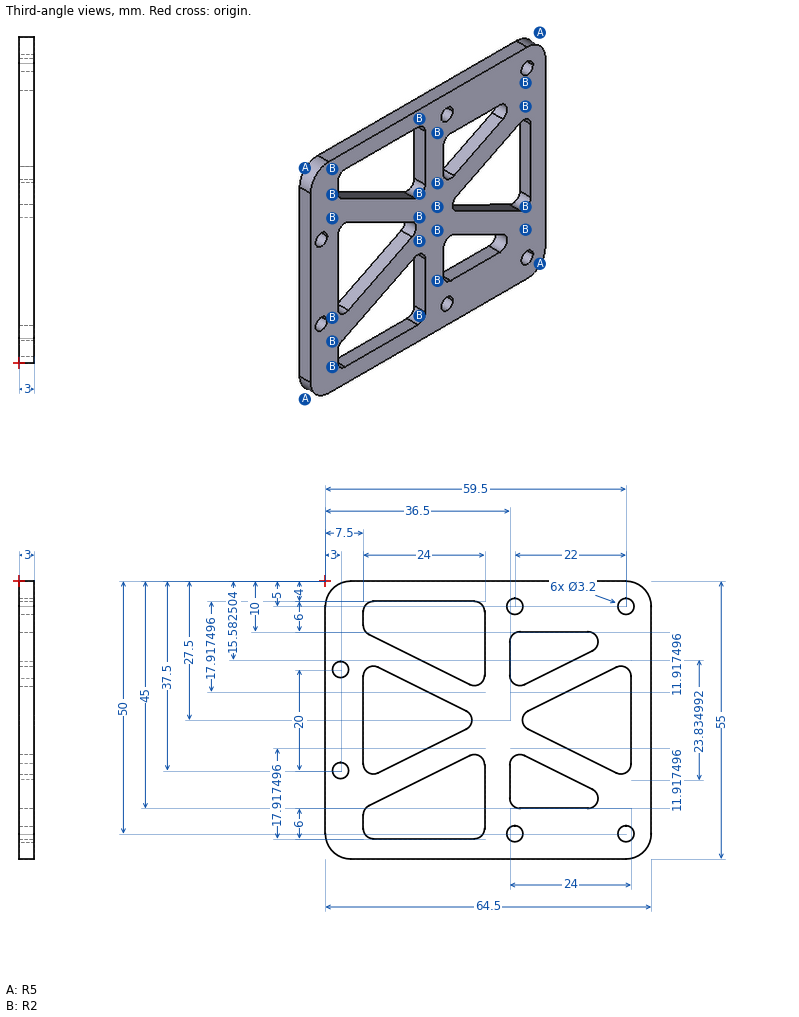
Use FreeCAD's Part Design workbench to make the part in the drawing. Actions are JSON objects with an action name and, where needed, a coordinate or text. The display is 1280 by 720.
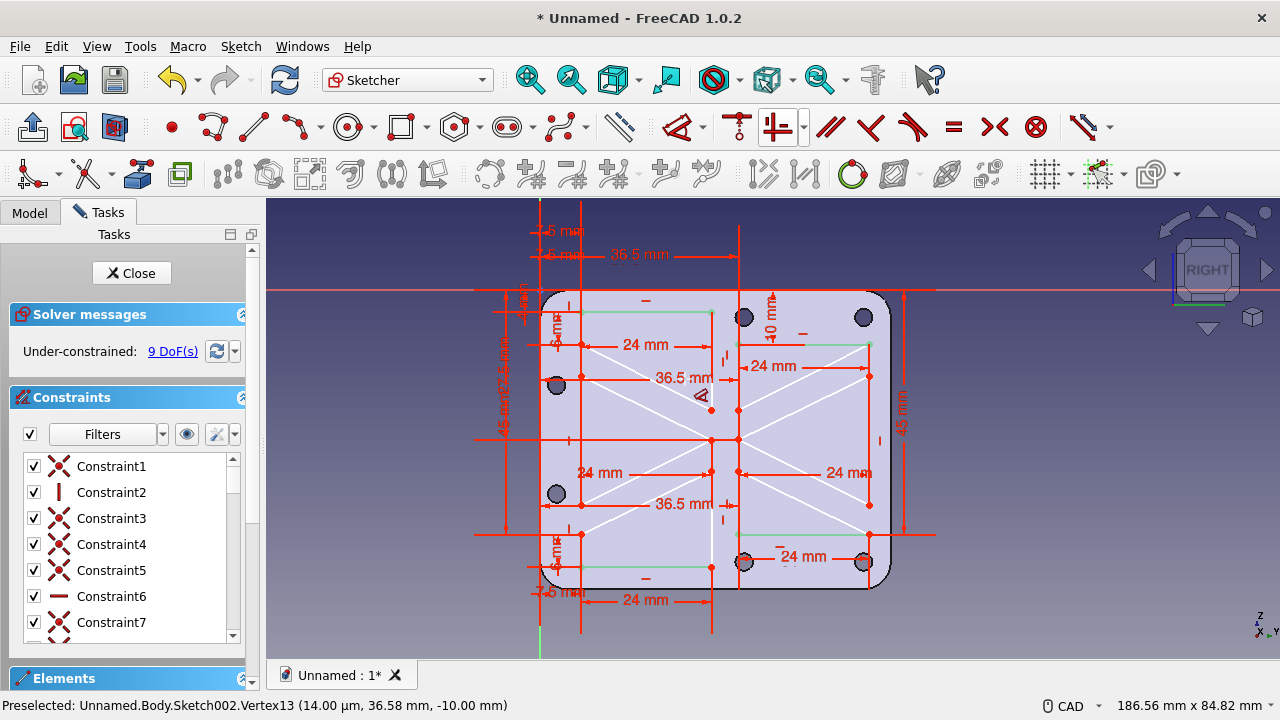
{"action": "left_click", "coordinate": [712, 440]}
{"action": "left_click", "coordinate": [482, 331]}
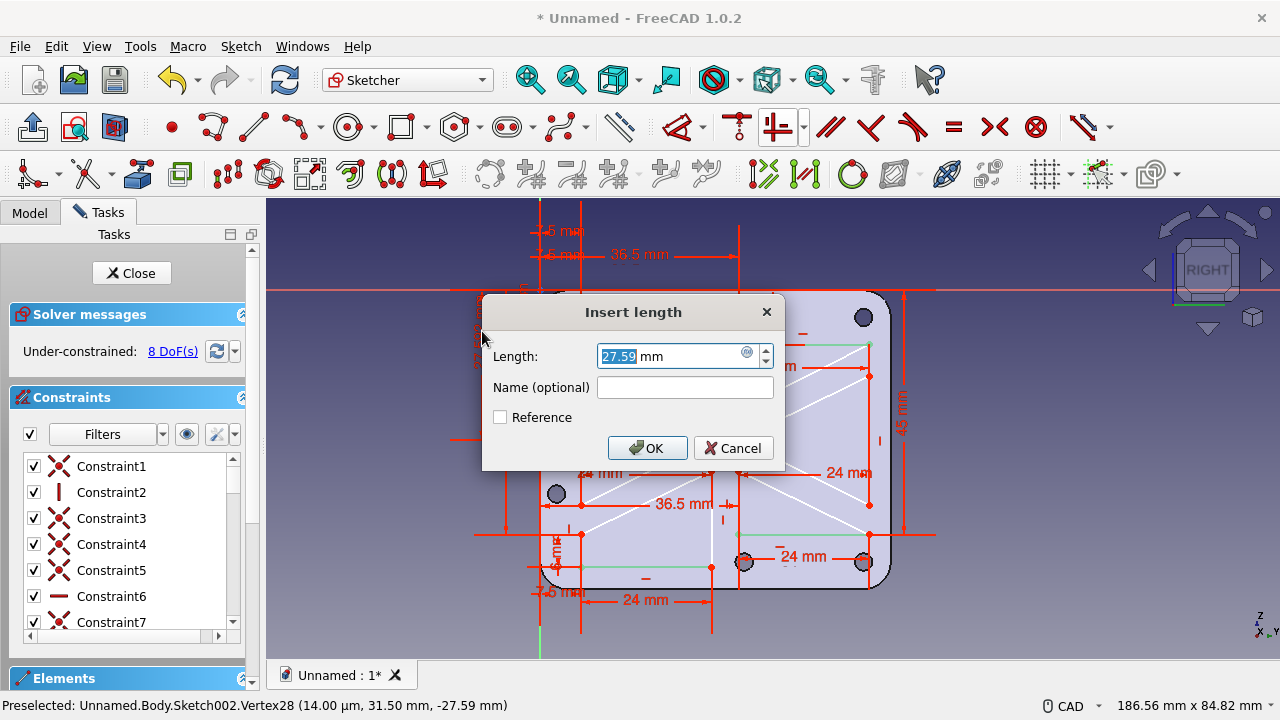
{"action": "type", "text": "27.5"}
{"action": "key", "text": "Return"}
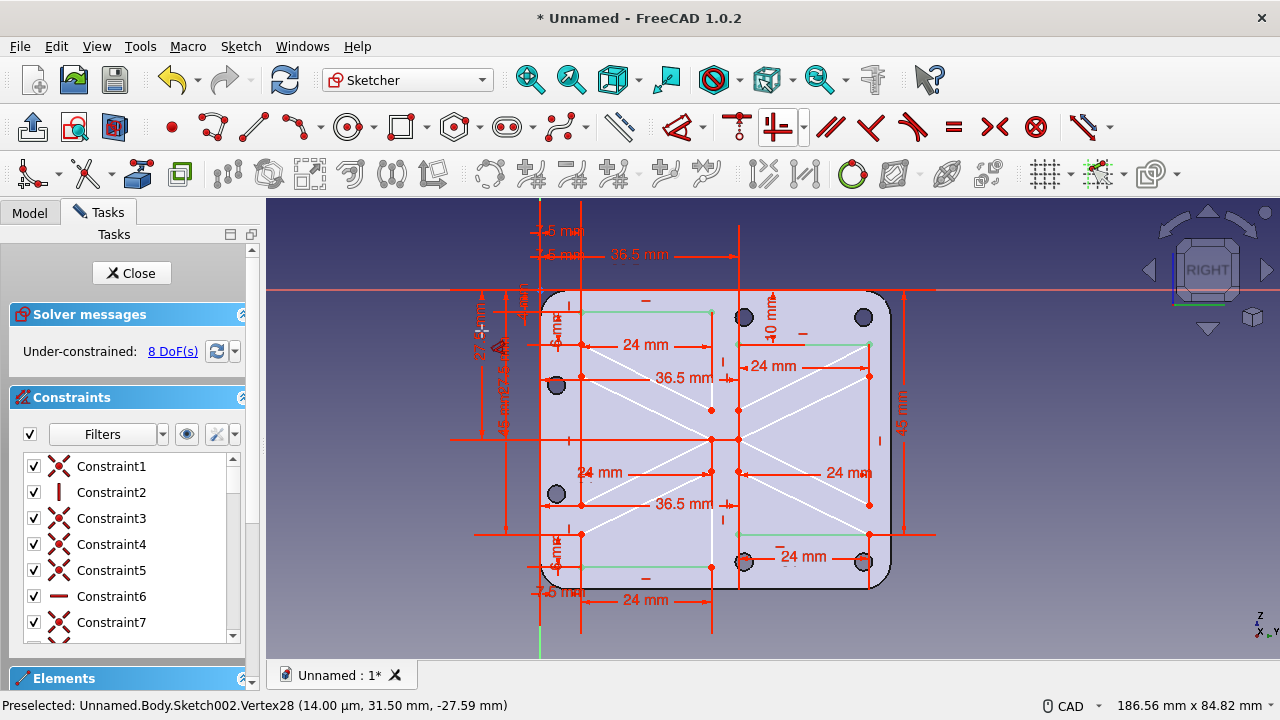
{"action": "left_click", "coordinate": [869, 415]}
{"action": "left_click", "coordinate": [903, 441]}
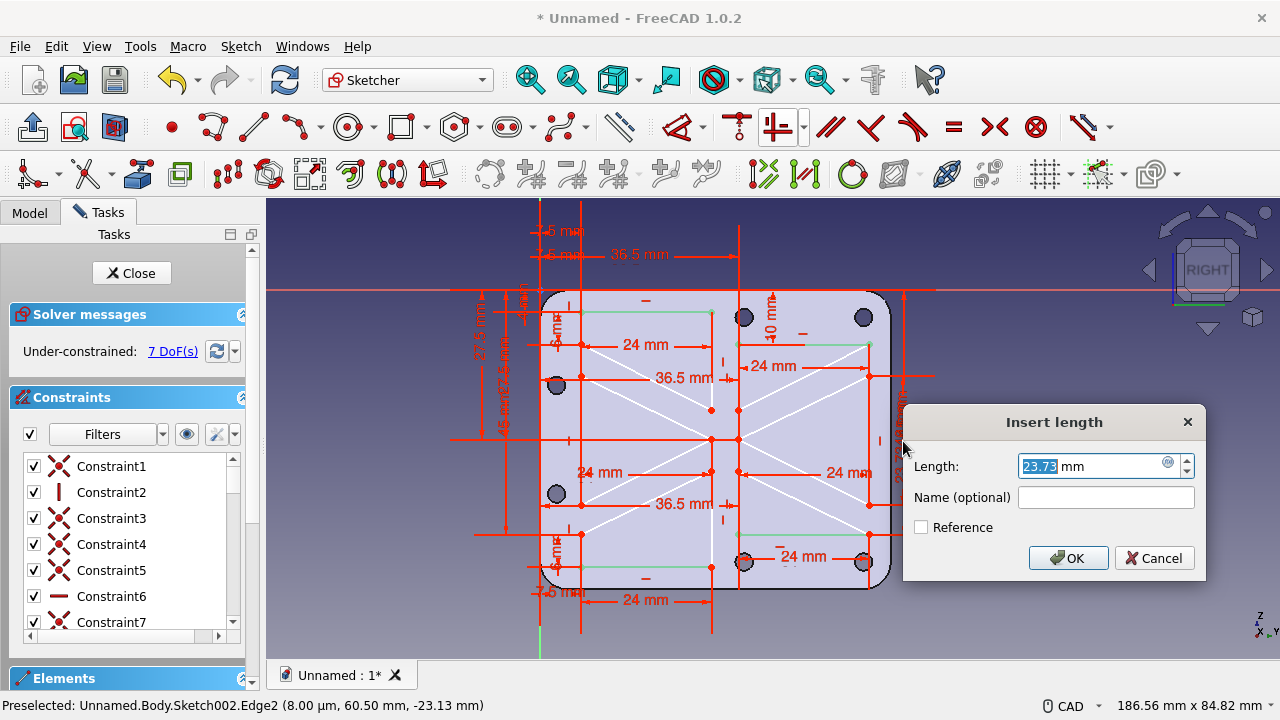
{"action": "type", "text": "23.834992"}
{"action": "key", "text": "Return"}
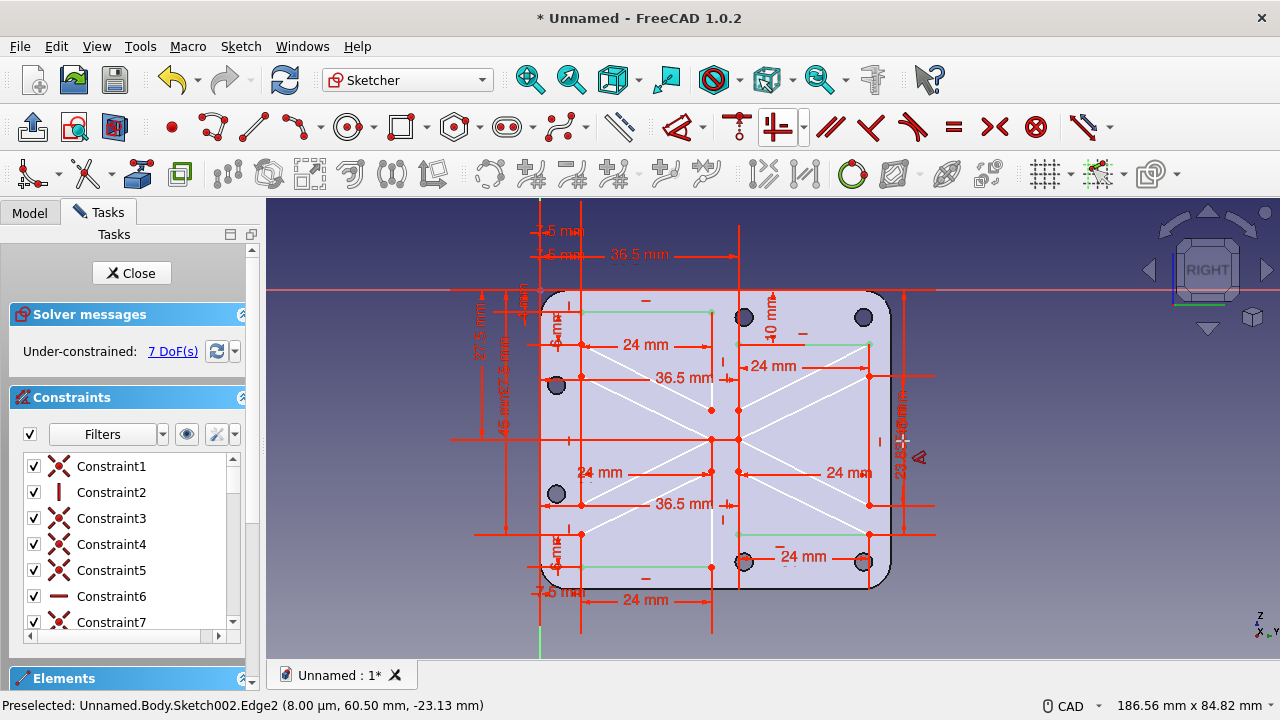
{"action": "left_click", "coordinate": [739, 516]}
{"action": "left_click", "coordinate": [773, 503]}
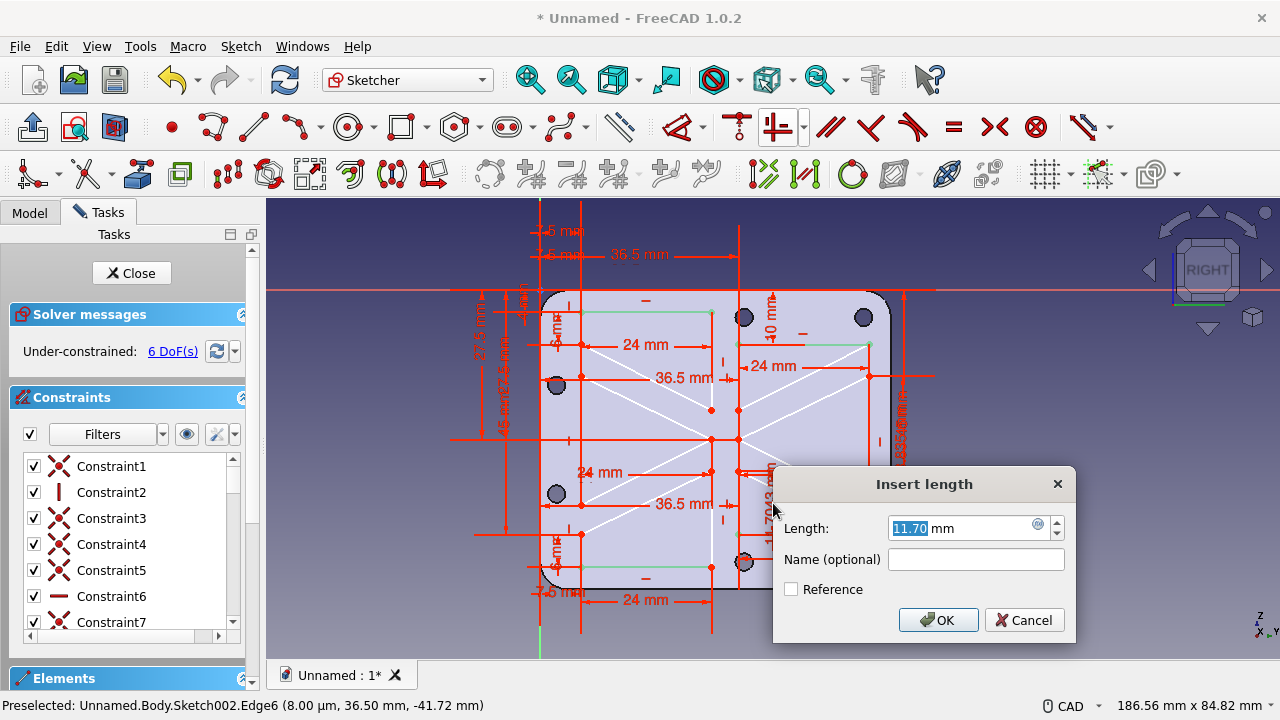
{"action": "type", "text": "11.917496"}
{"action": "key", "text": "Return"}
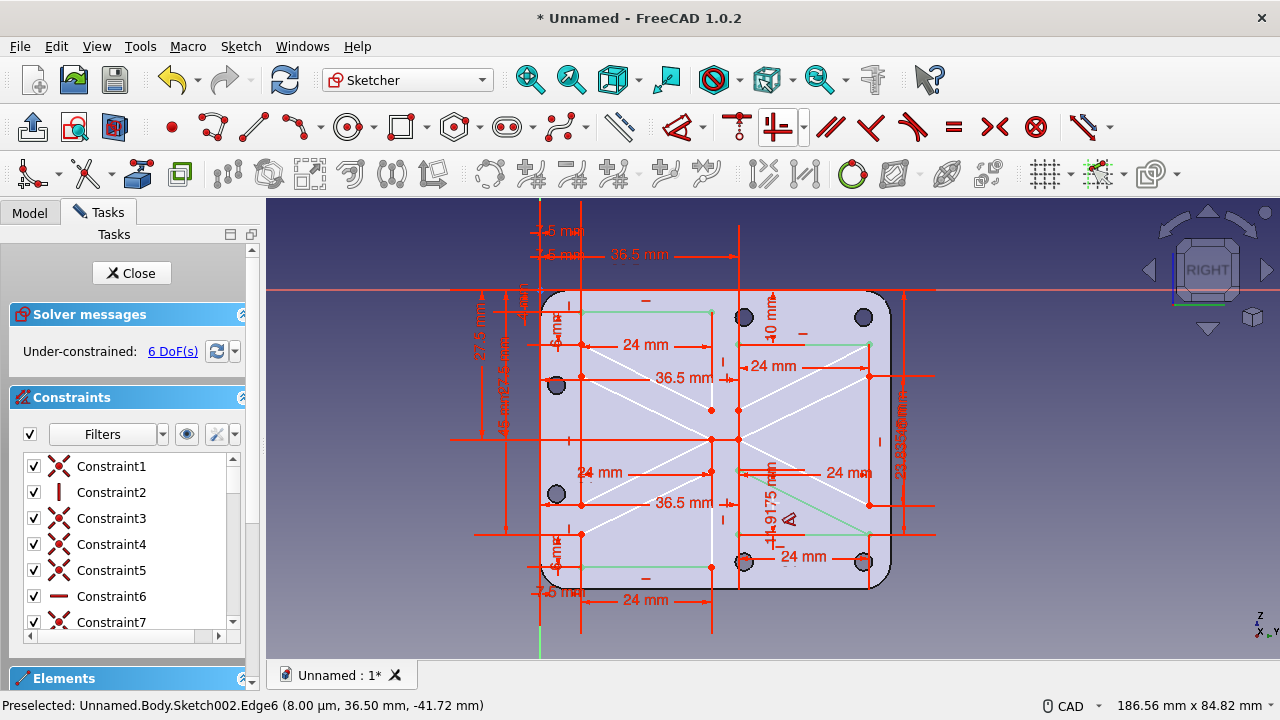
{"action": "left_click", "coordinate": [739, 391]}
{"action": "left_click", "coordinate": [869, 362]}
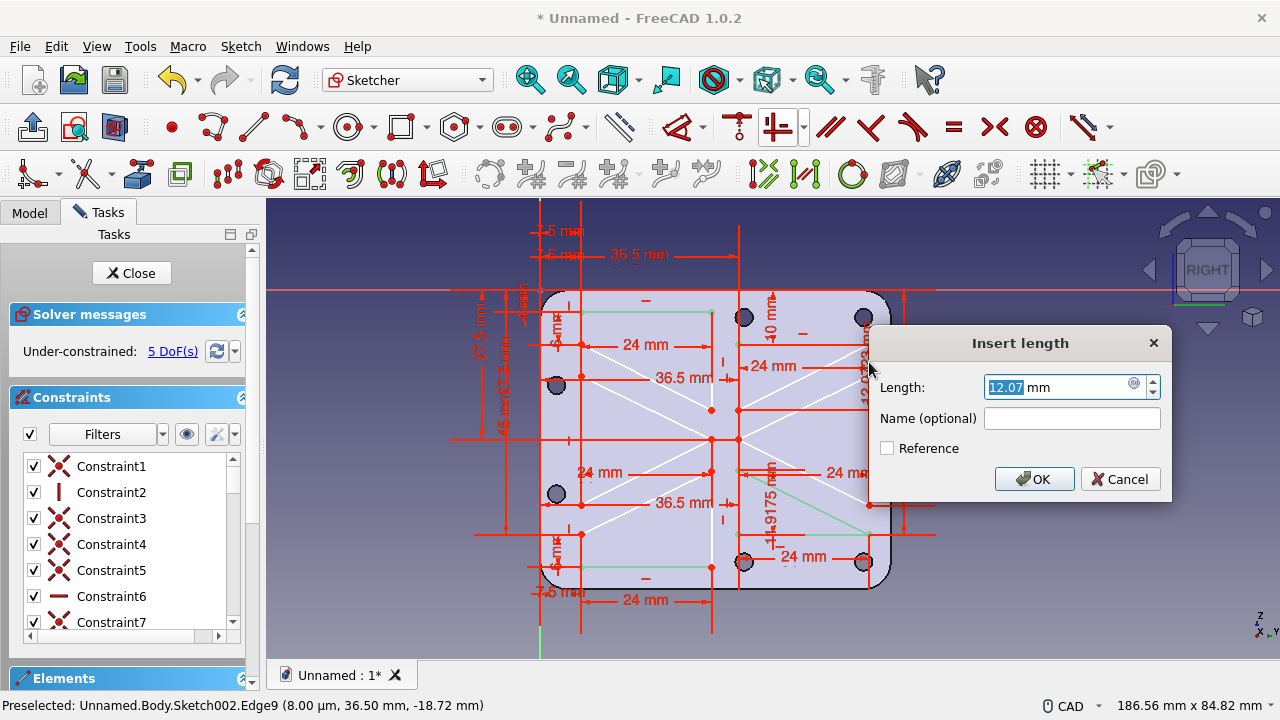
{"action": "type", "text": "11.917496"}
{"action": "key", "text": "Return"}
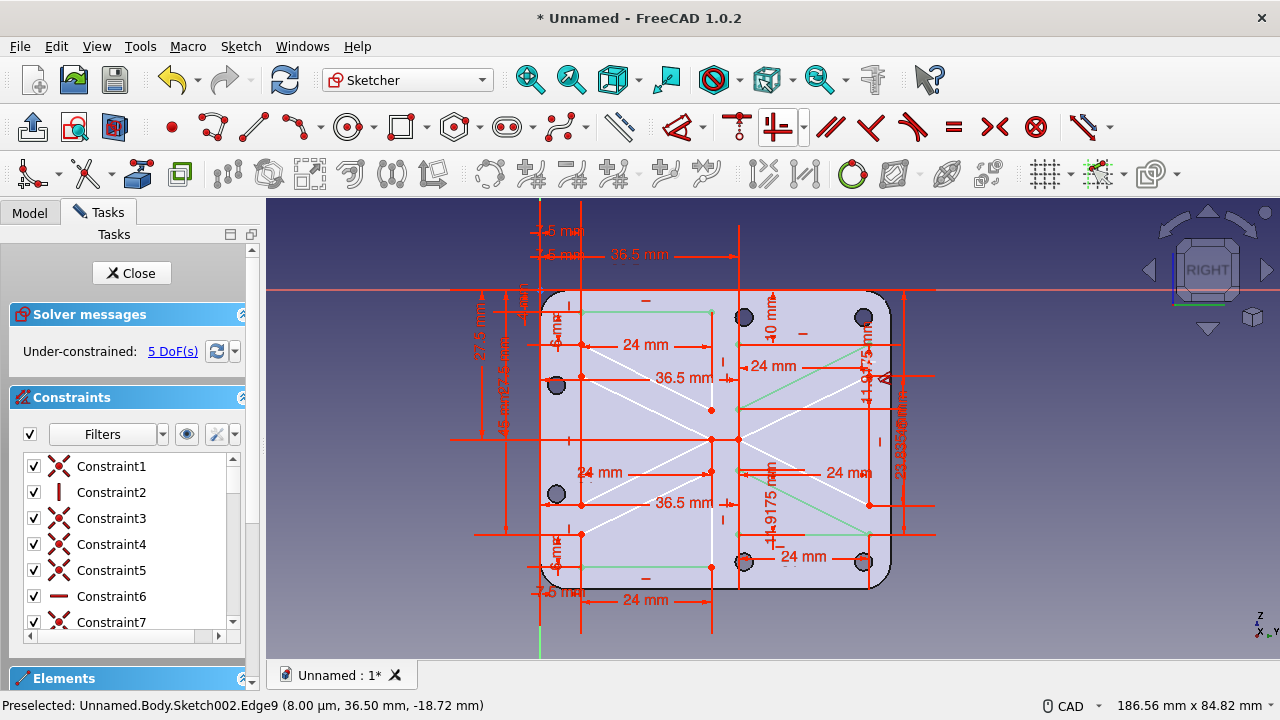
{"action": "left_click", "coordinate": [712, 341]}
{"action": "left_click", "coordinate": [678, 327]}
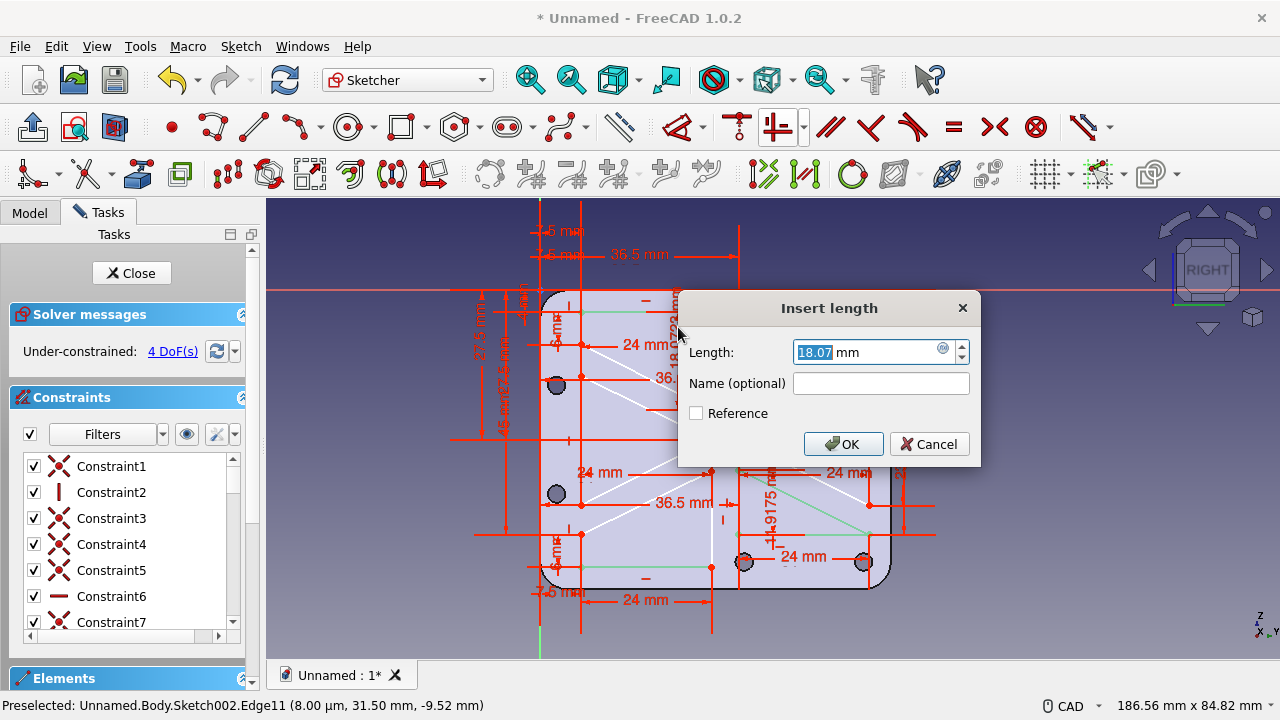
{"action": "type", "text": "17.917496"}
{"action": "key", "text": "Return"}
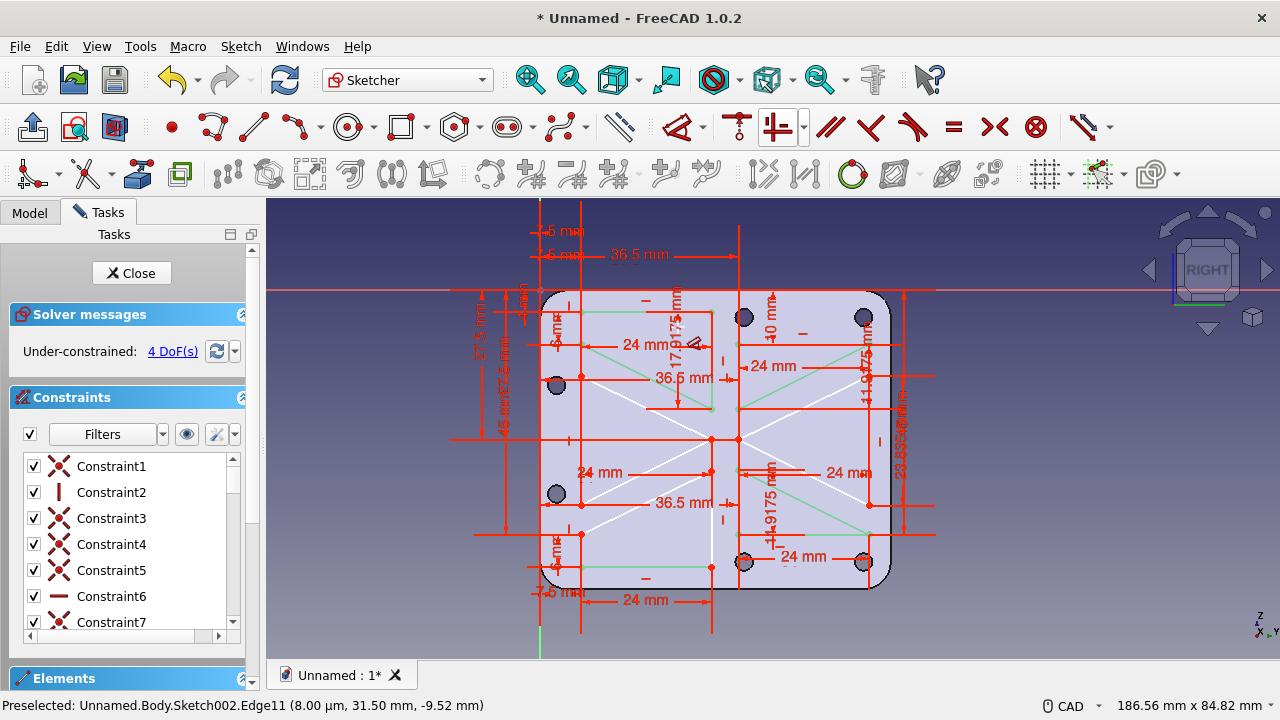
{"action": "left_click", "coordinate": [581, 467]}
{"action": "left_click", "coordinate": [615, 441]}